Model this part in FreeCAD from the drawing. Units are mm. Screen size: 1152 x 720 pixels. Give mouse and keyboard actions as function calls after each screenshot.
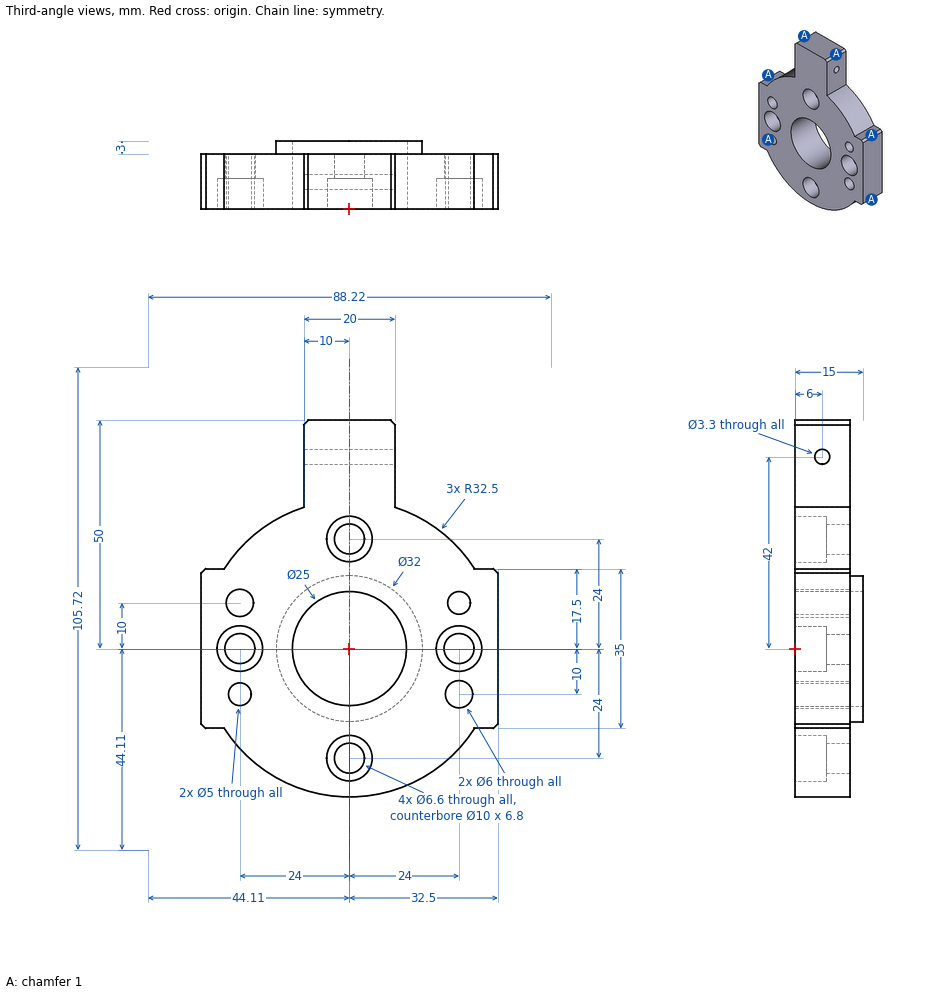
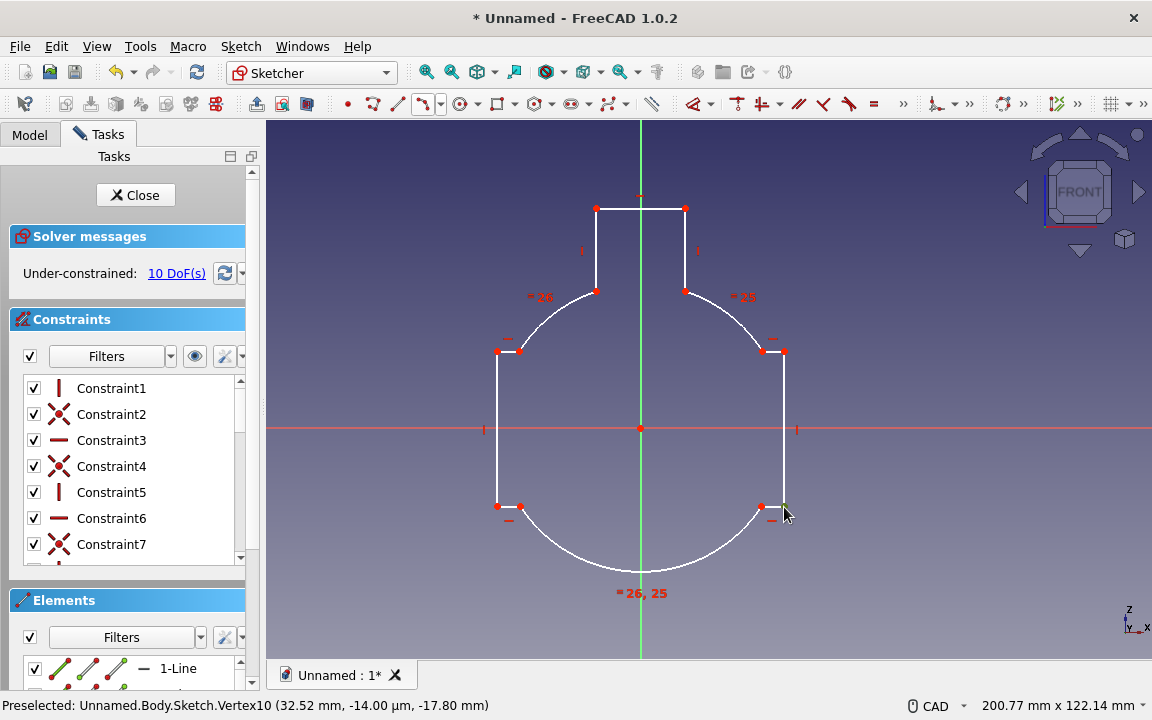
click(497, 507)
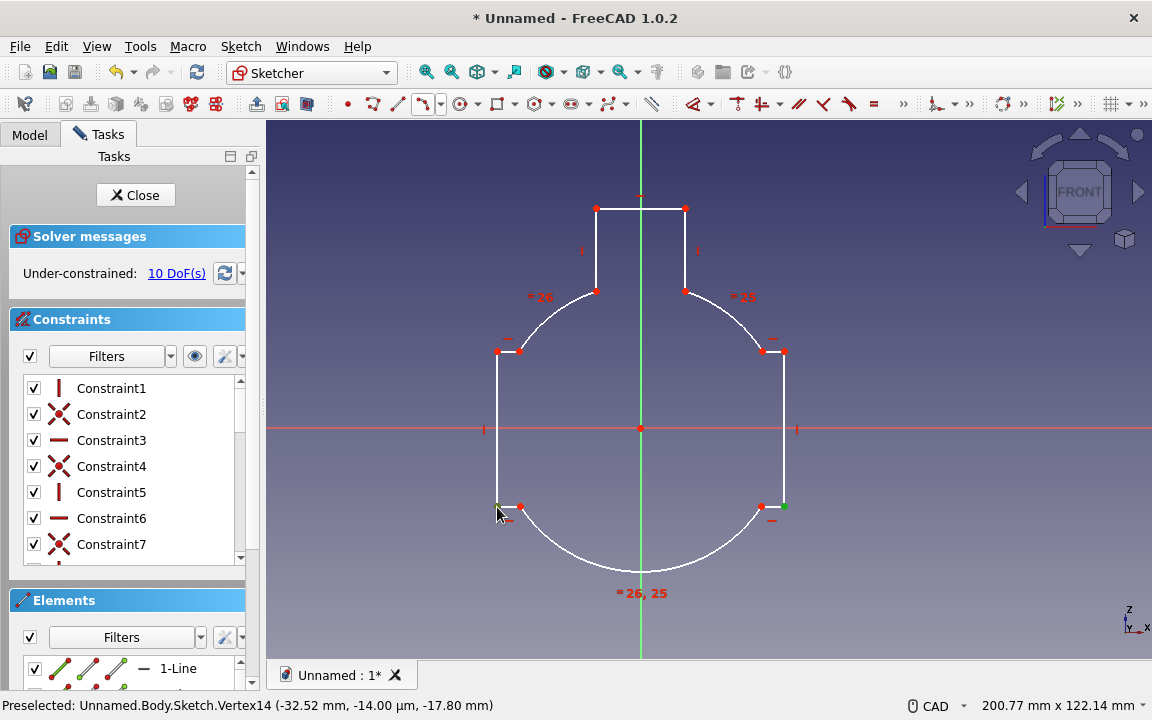
click(641, 528)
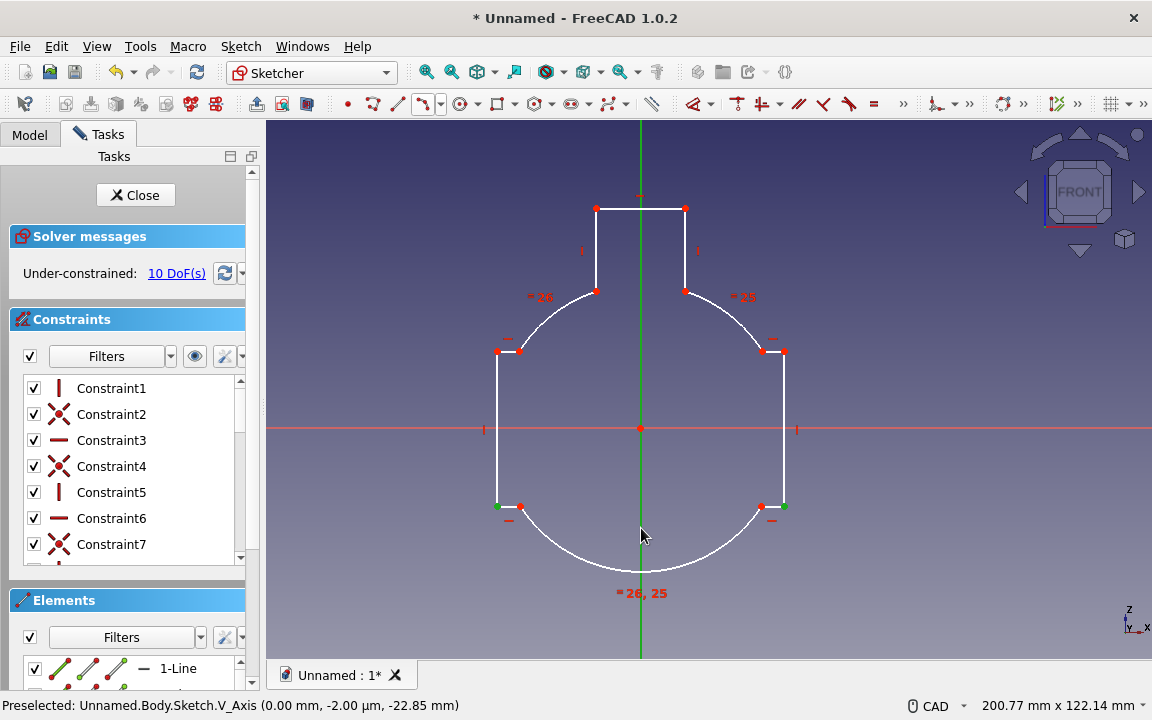
key(s)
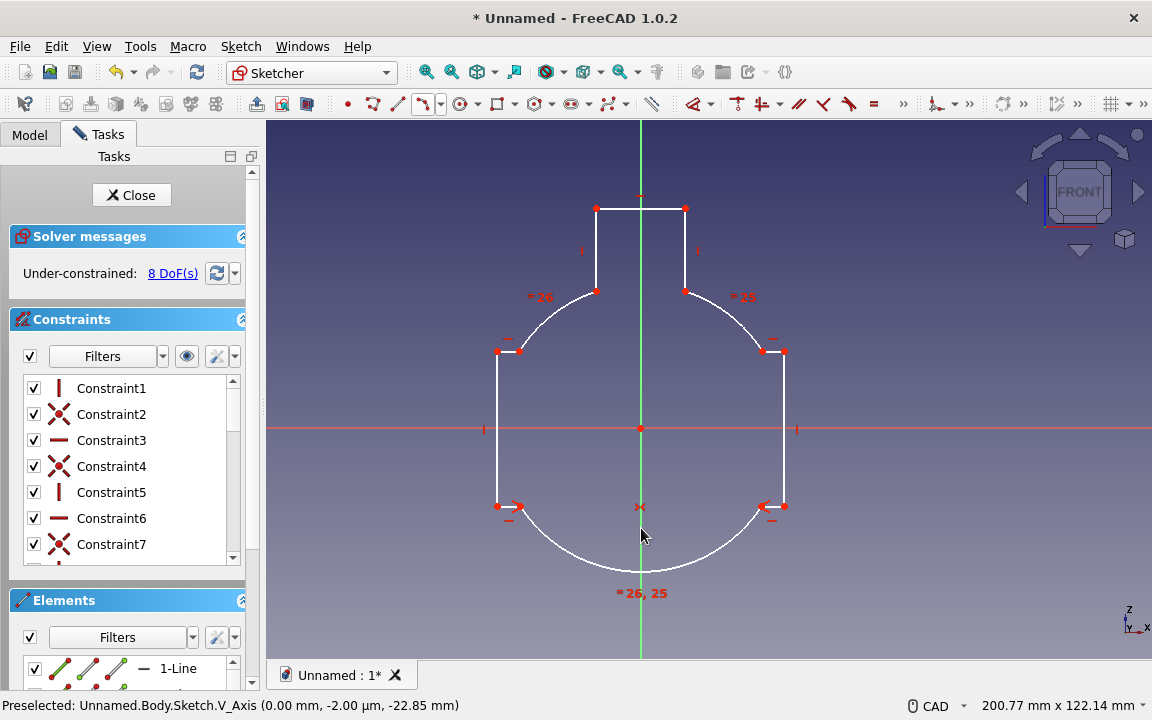
click(692, 104)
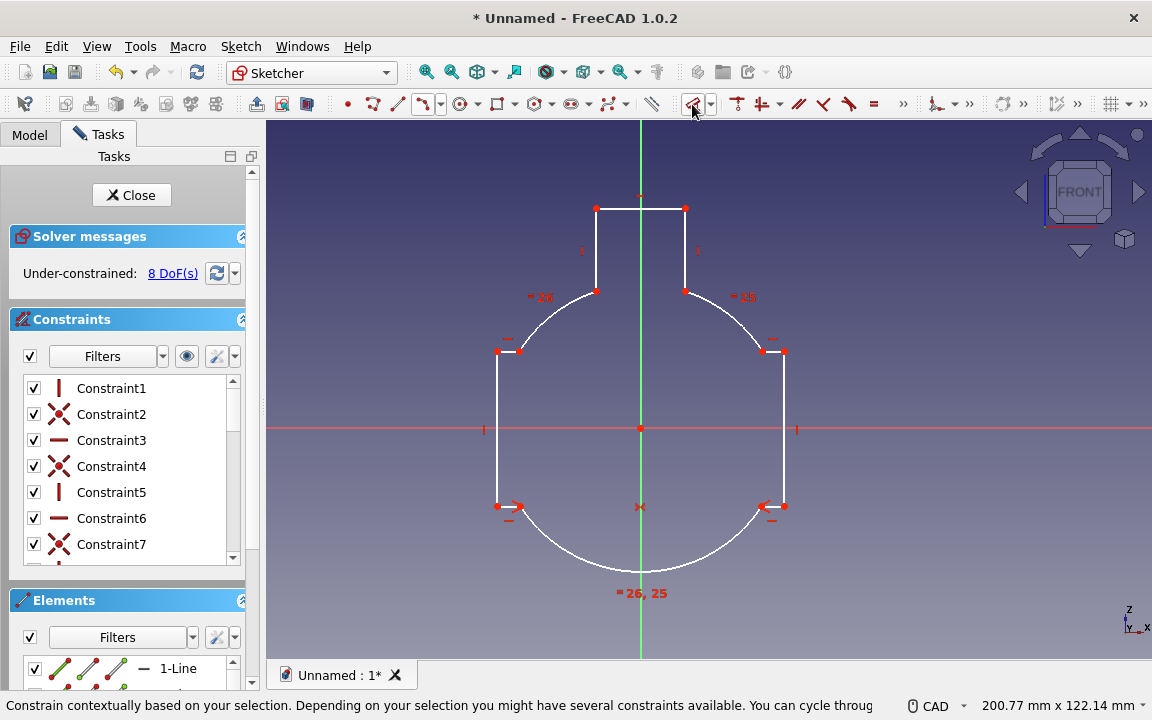
click(744, 328)
click(767, 306)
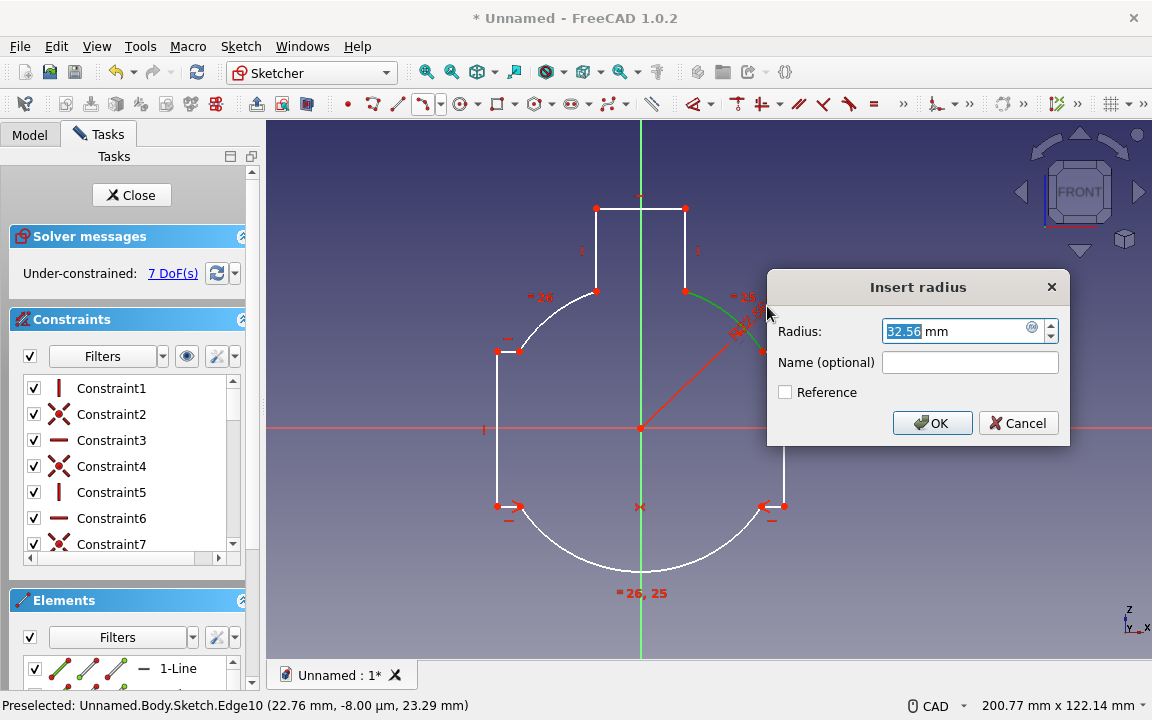
text(32.5)
key(Return)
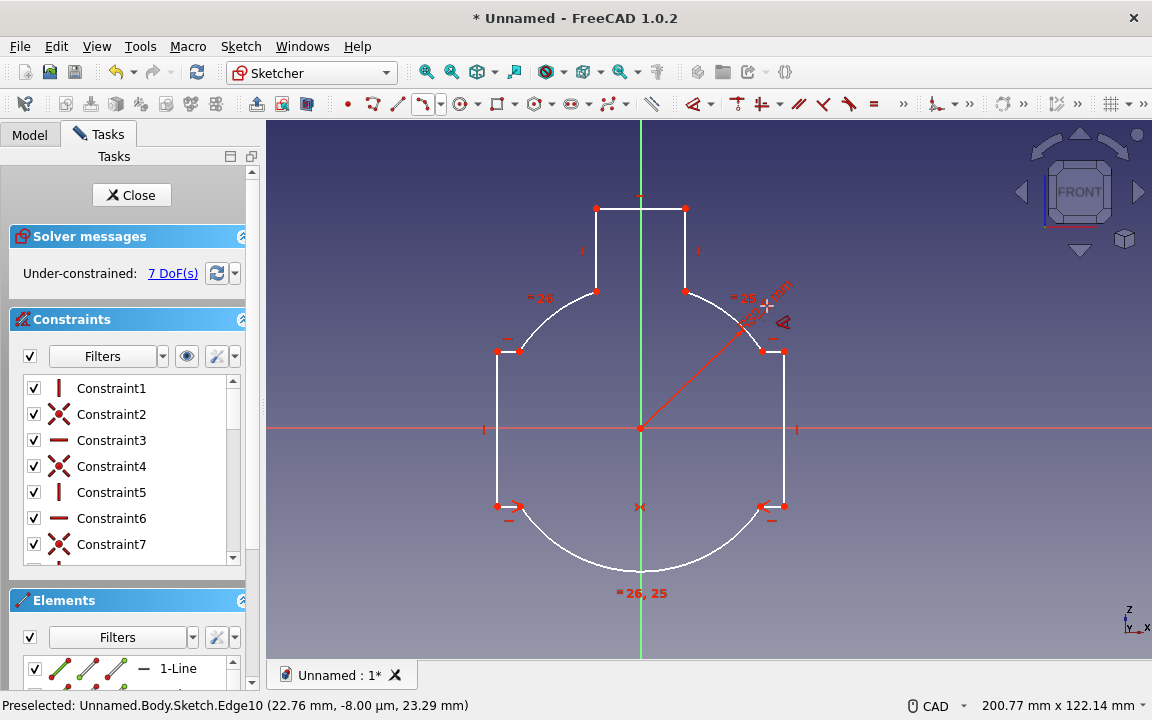
click(623, 209)
click(620, 175)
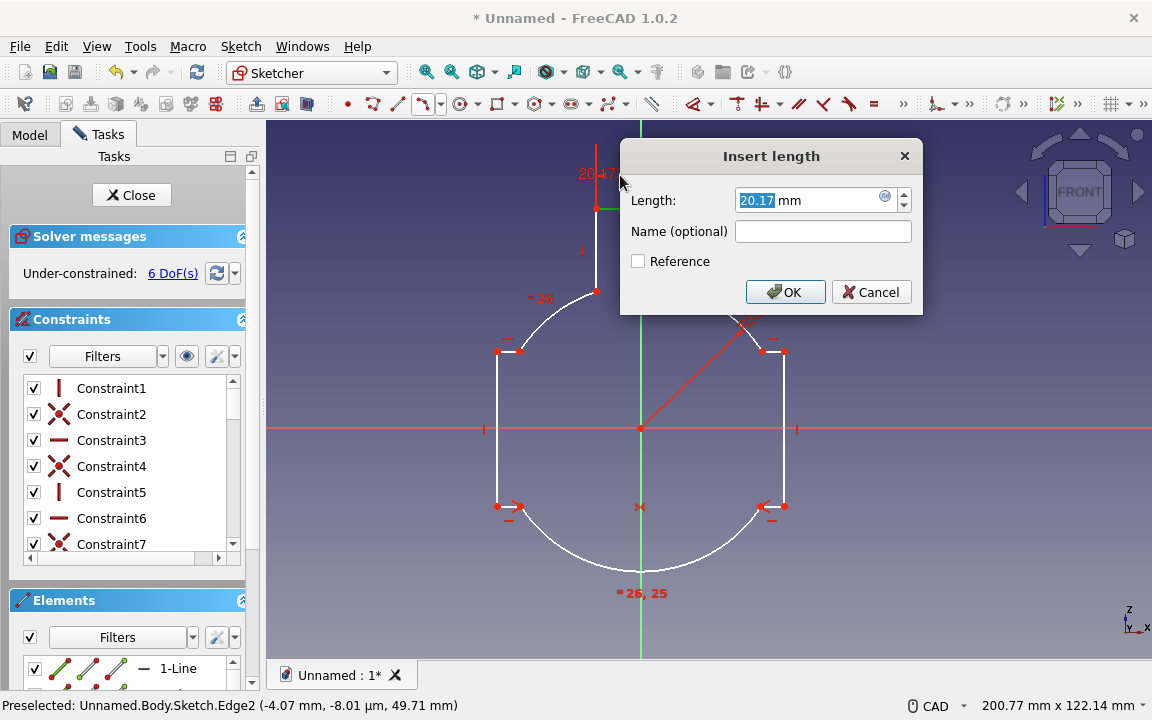
text(20)
key(Return)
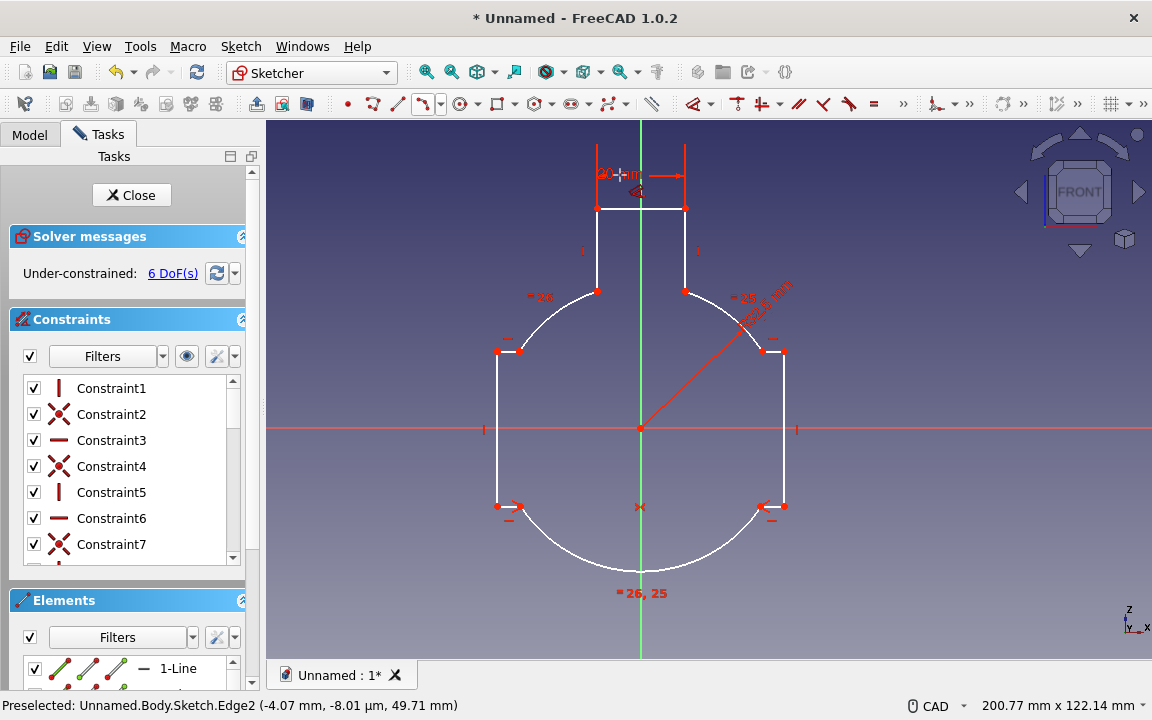
click(784, 398)
click(818, 394)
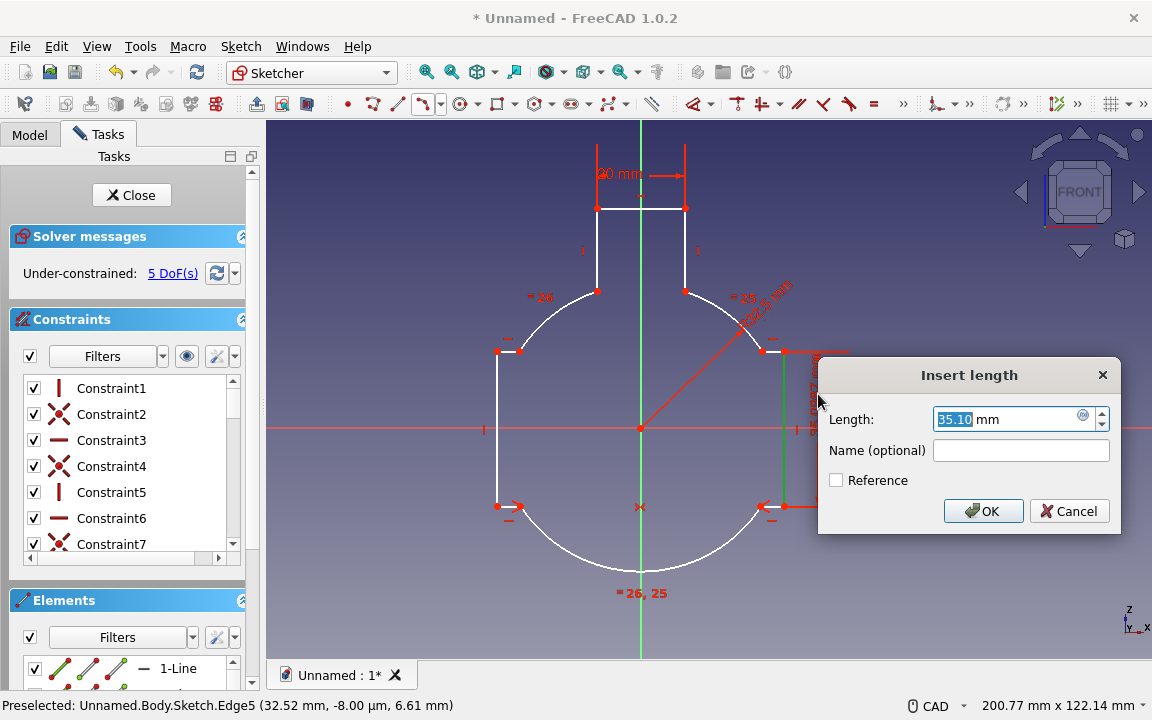
text(35)
key(Return)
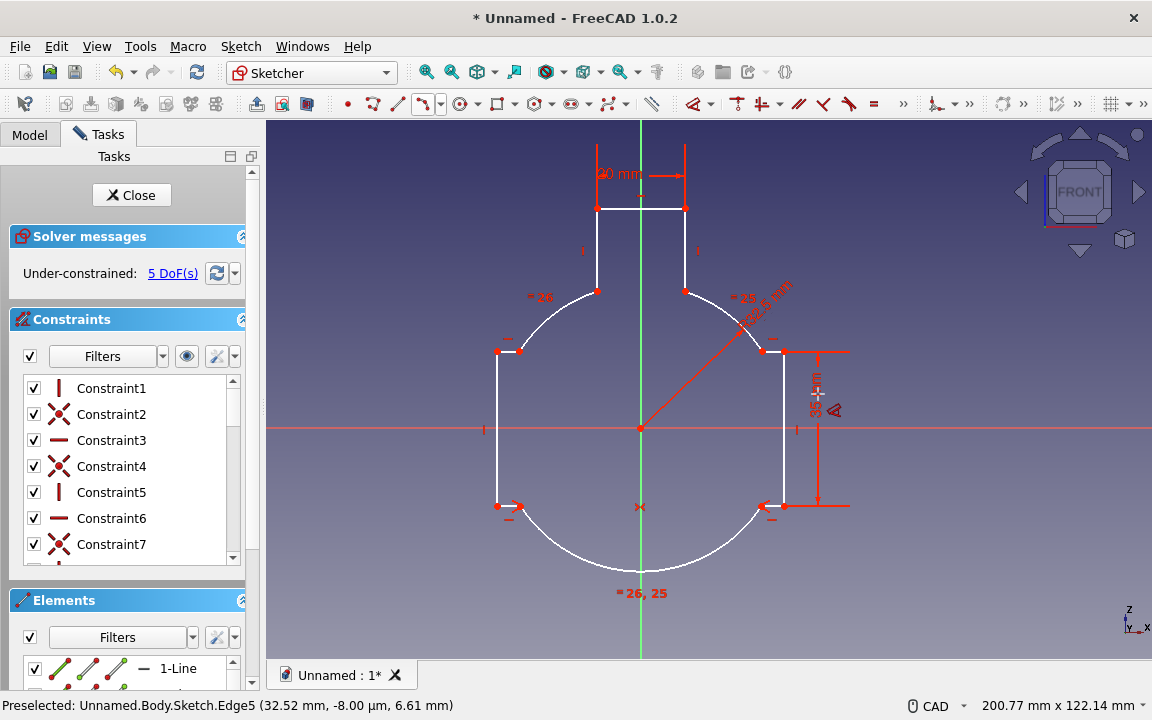
click(497, 460)
click(463, 393)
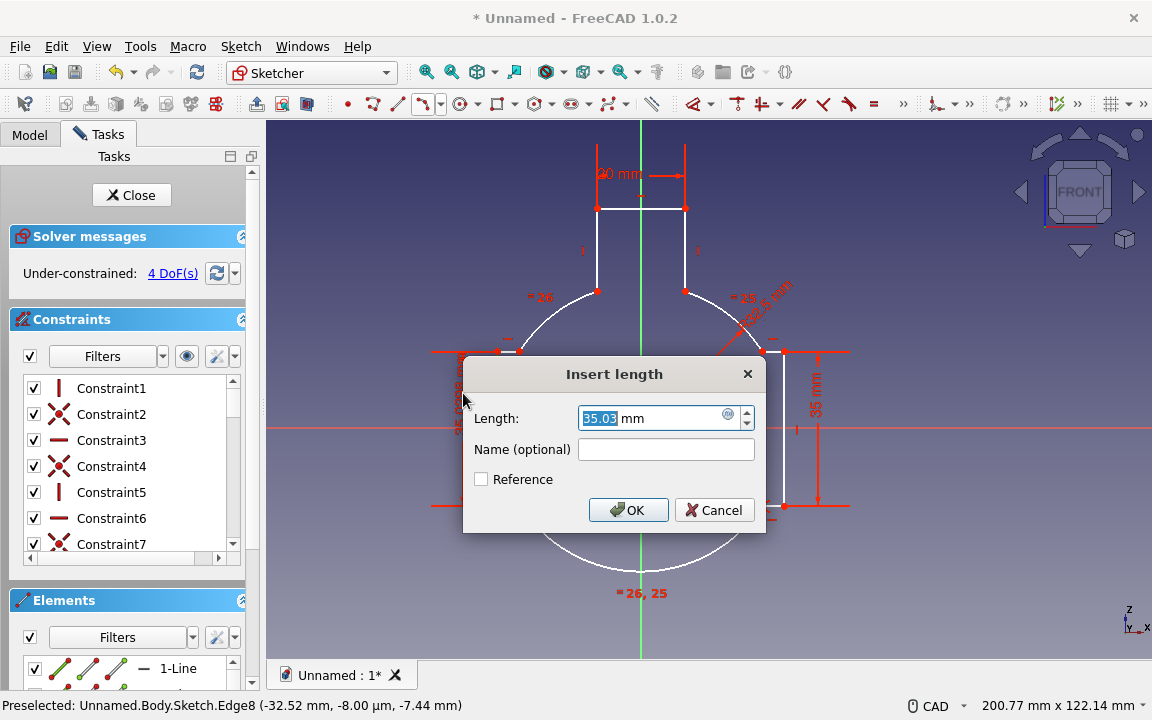
text(35)
key(Return)